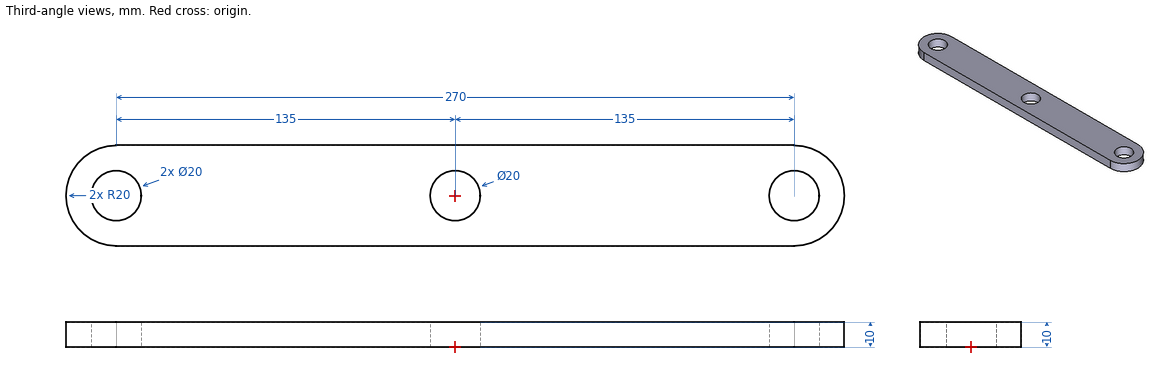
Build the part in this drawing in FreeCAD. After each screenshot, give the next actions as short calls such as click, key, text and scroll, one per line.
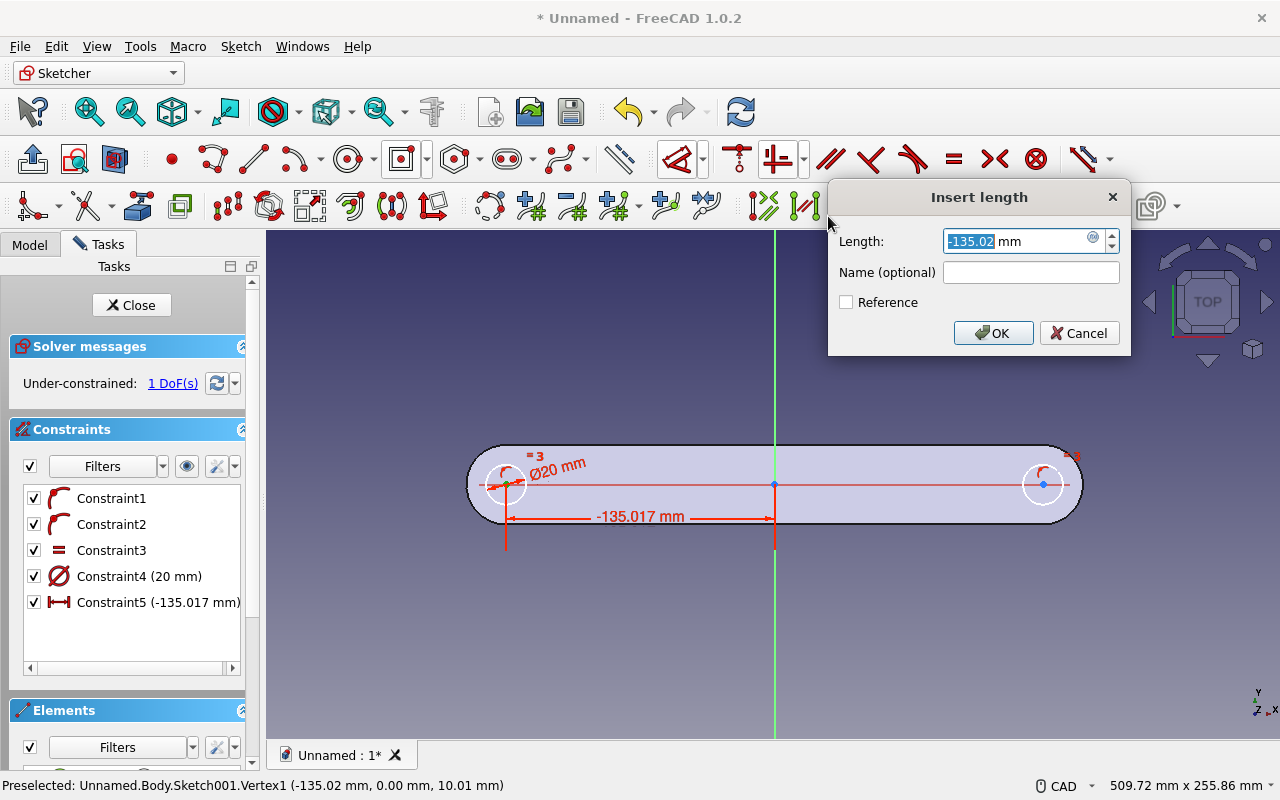
text(-135)
key(Return)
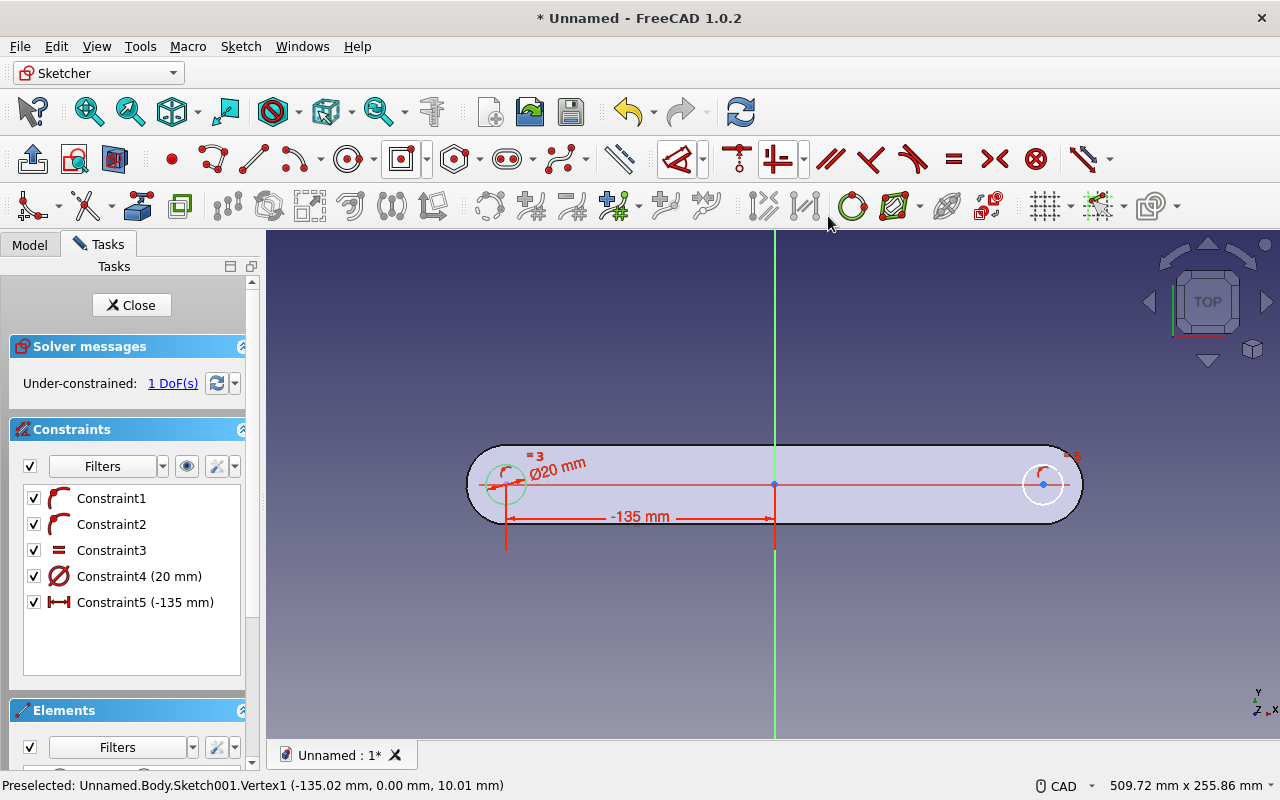
click(1043, 485)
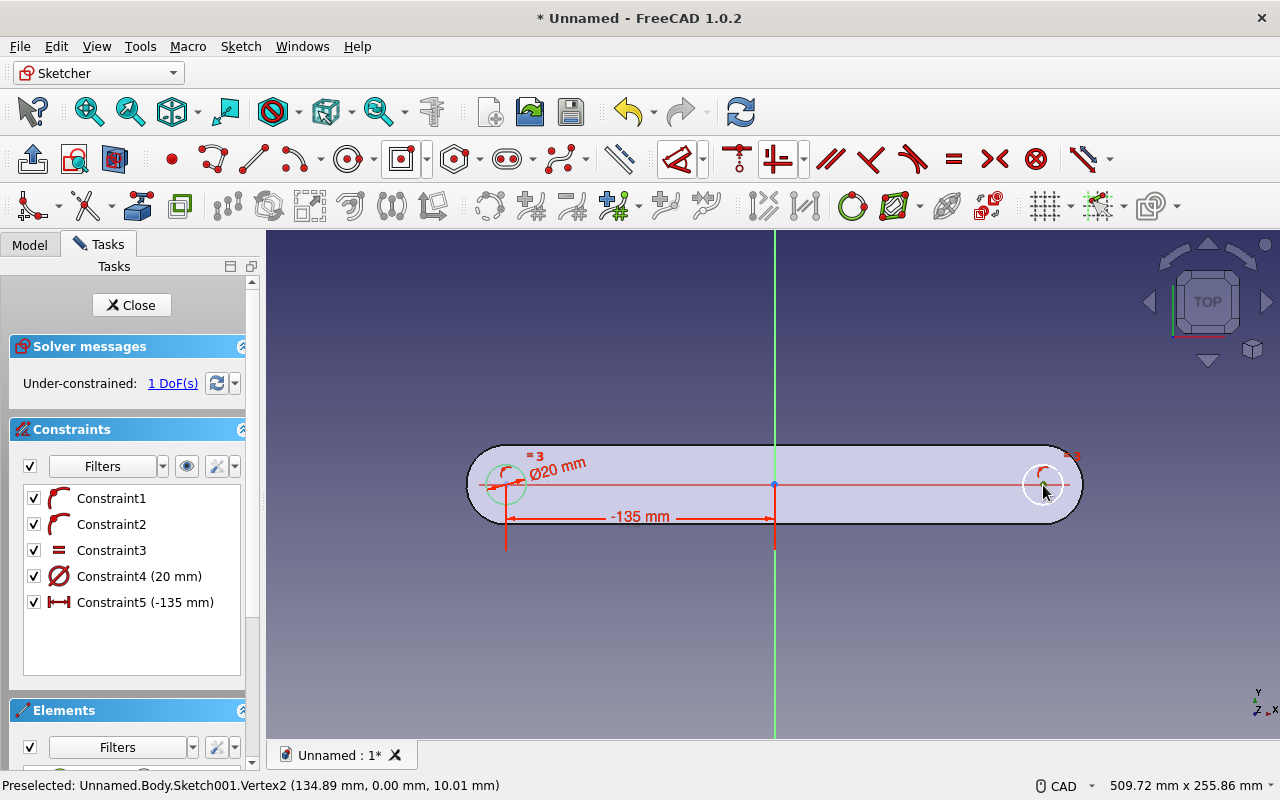
key(l)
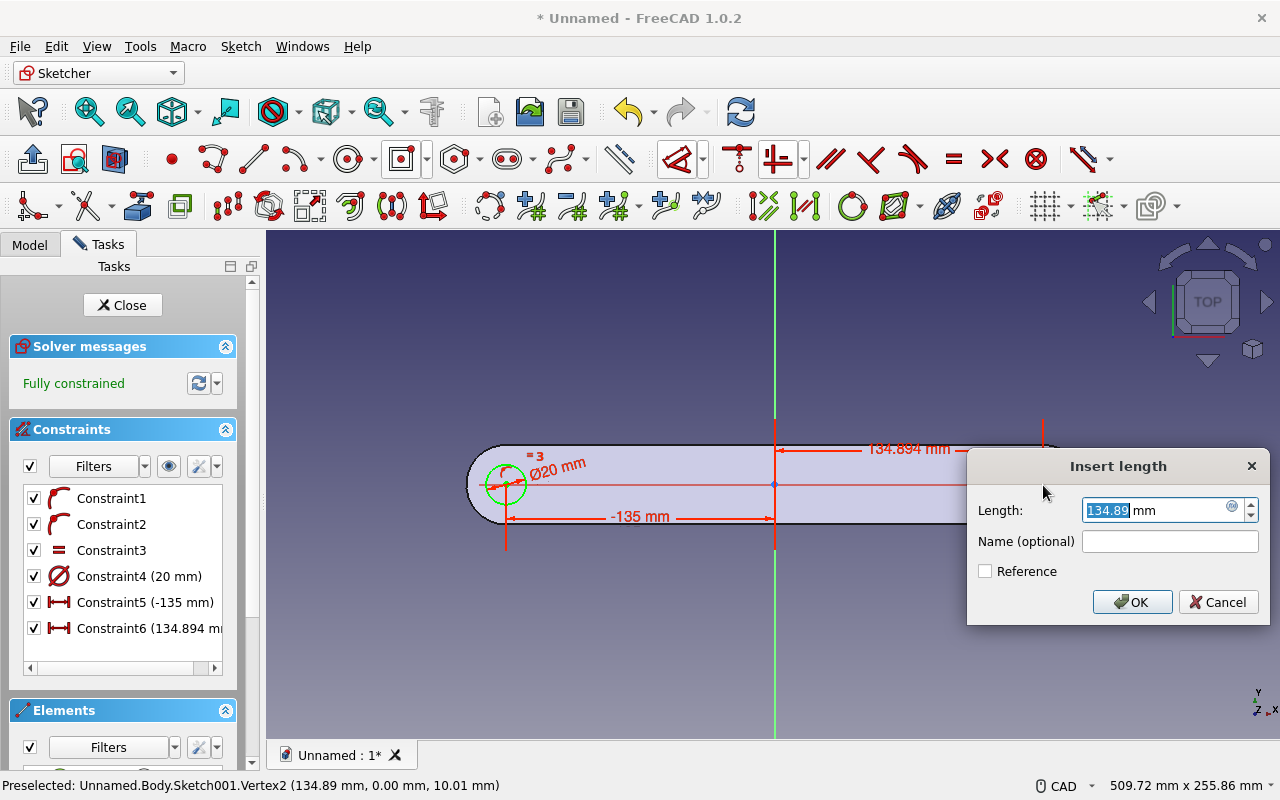
text(135)
key(Return)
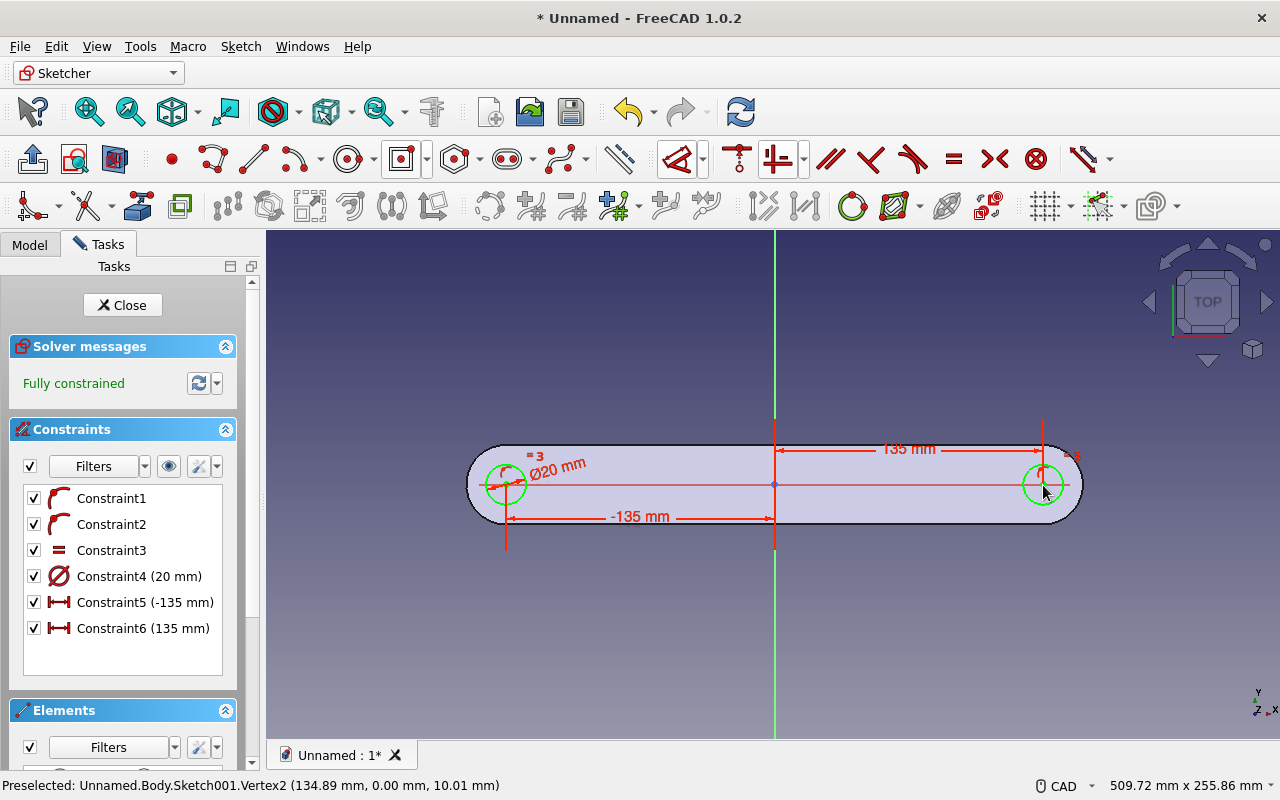
click(123, 305)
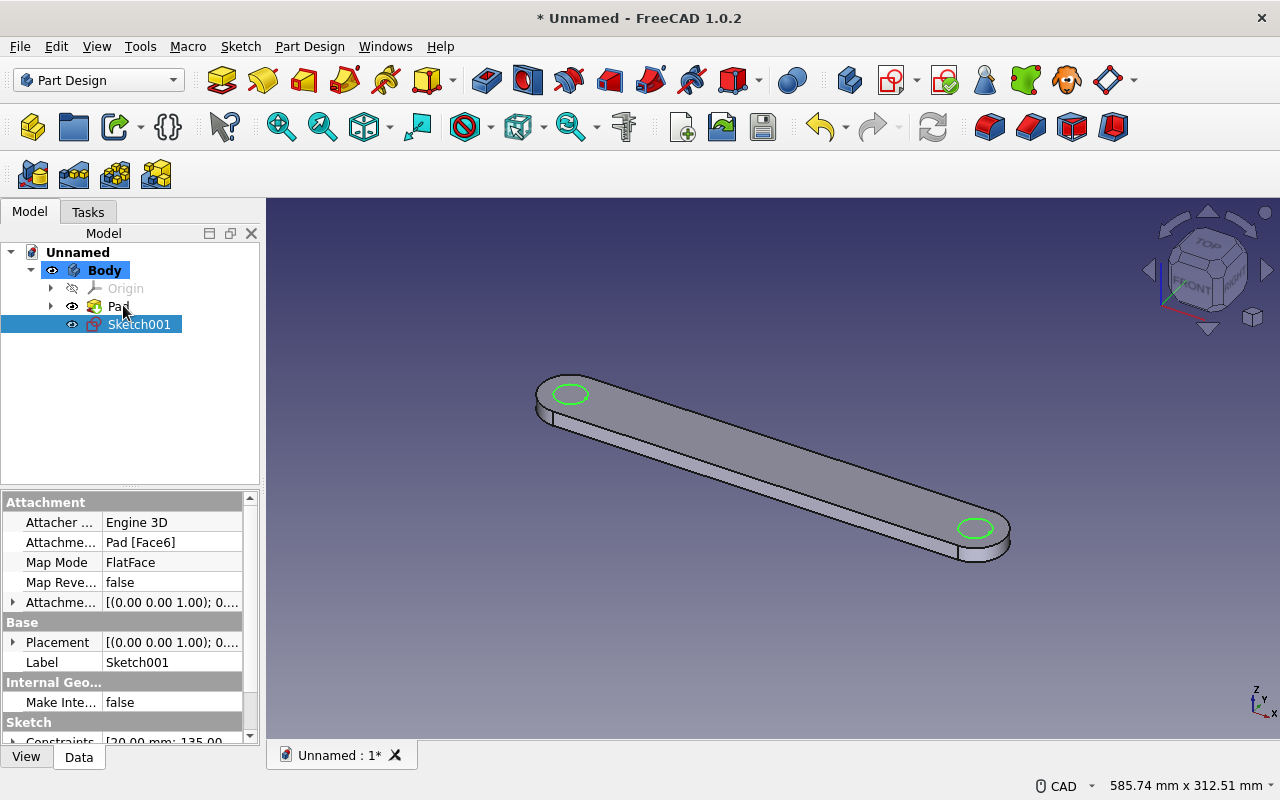
click(487, 80)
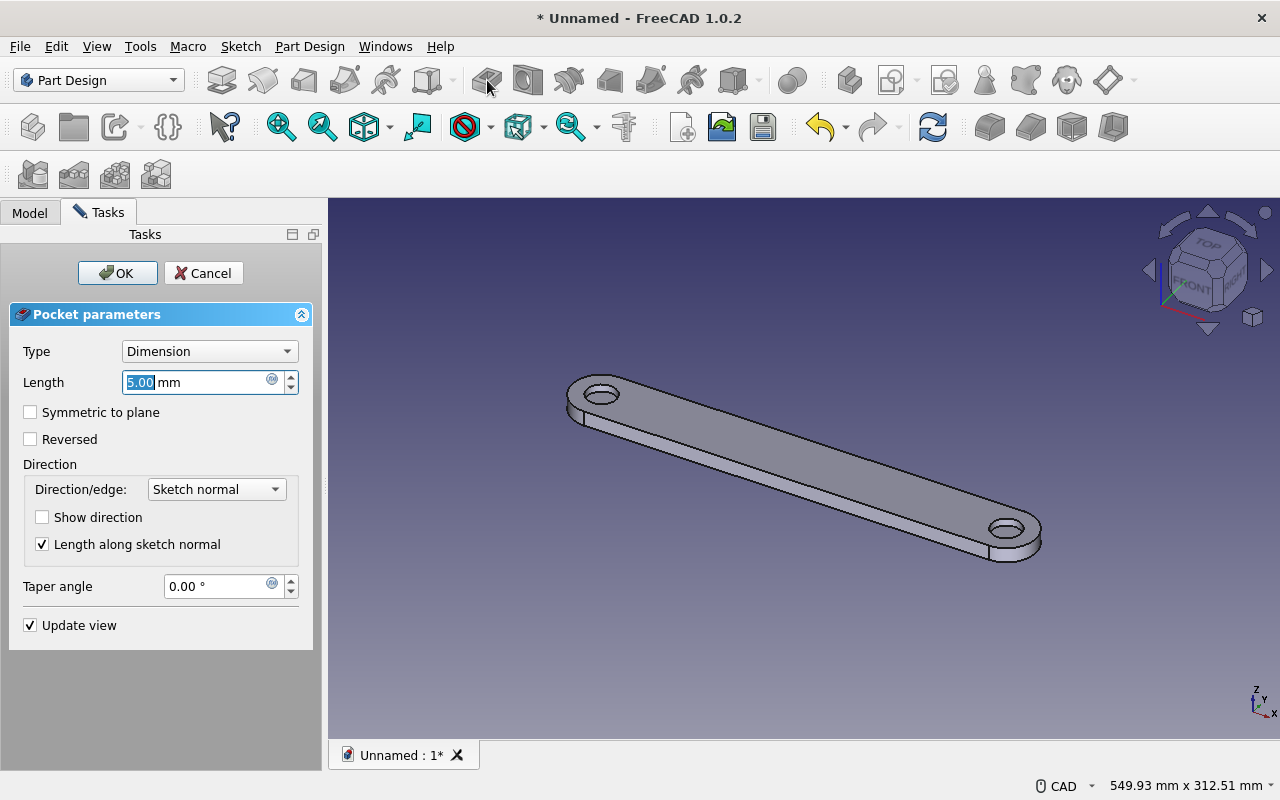
click(210, 352)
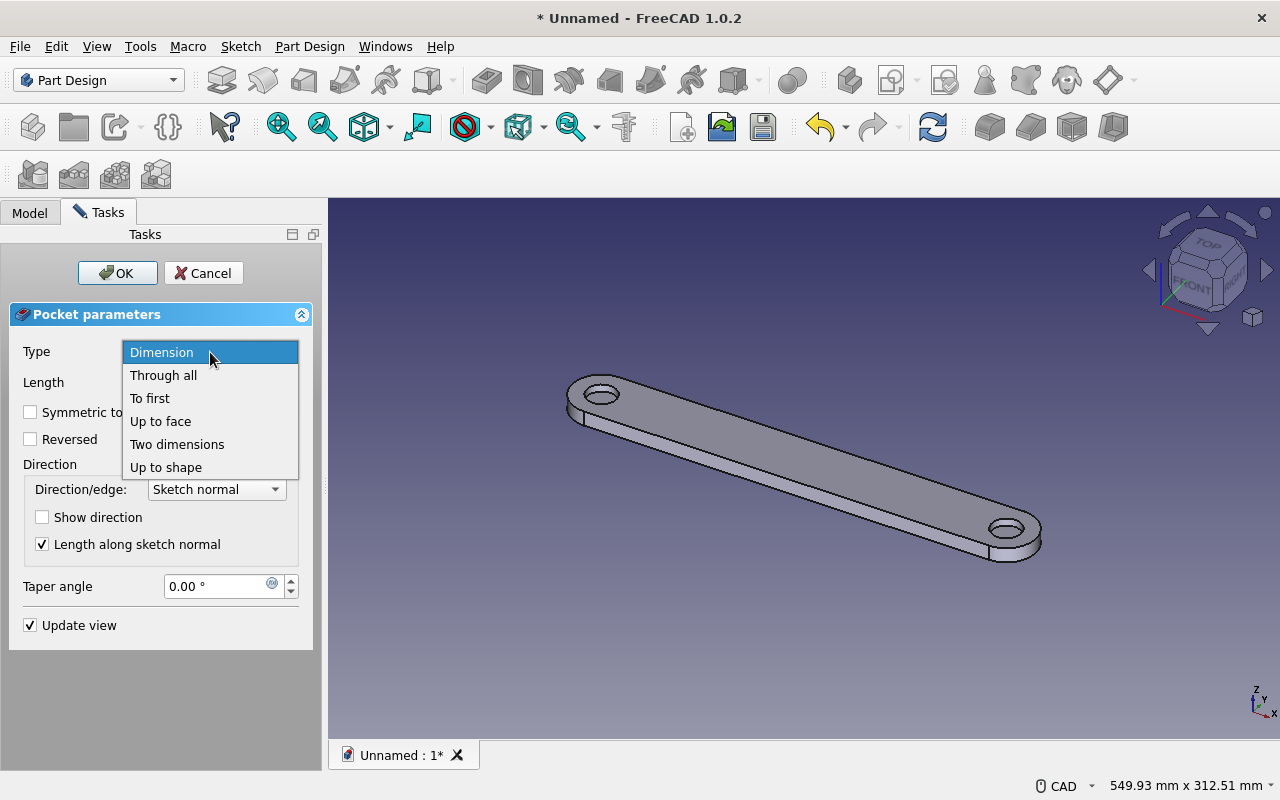
click(208, 376)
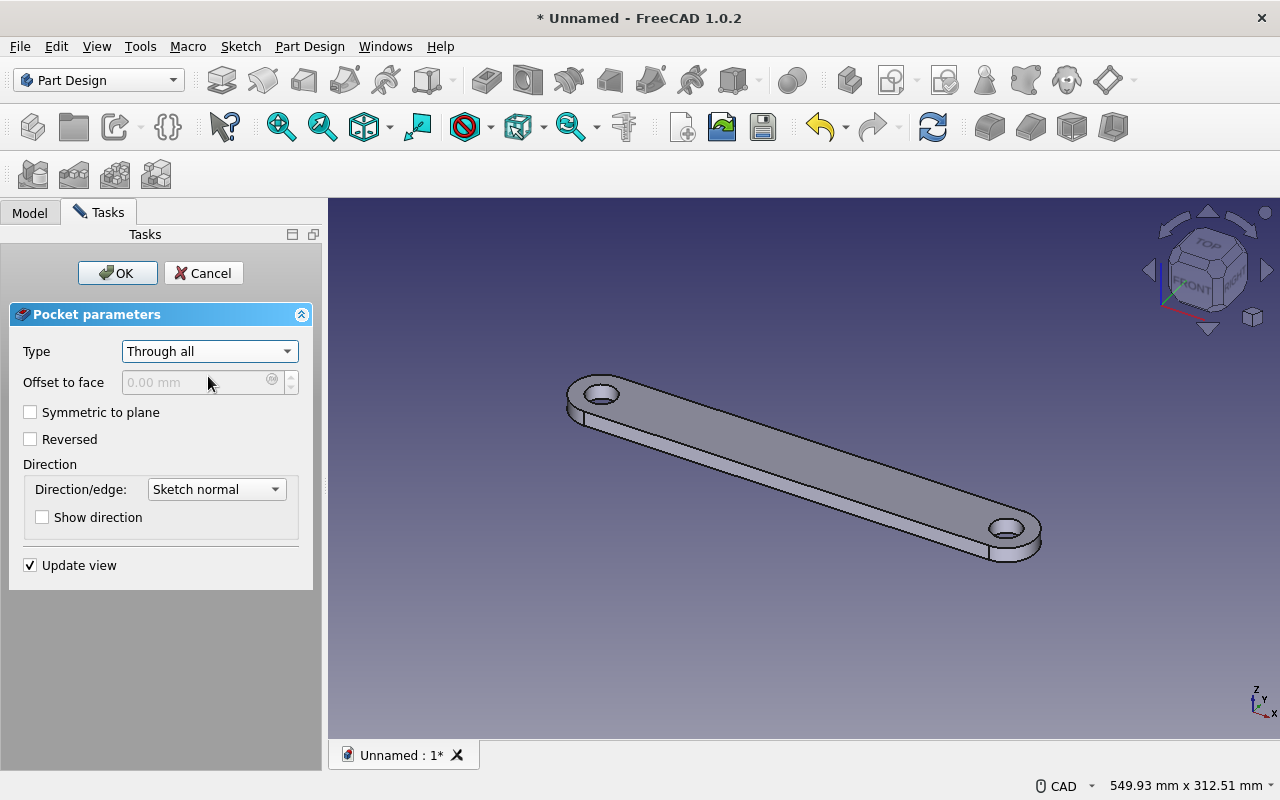
click(118, 273)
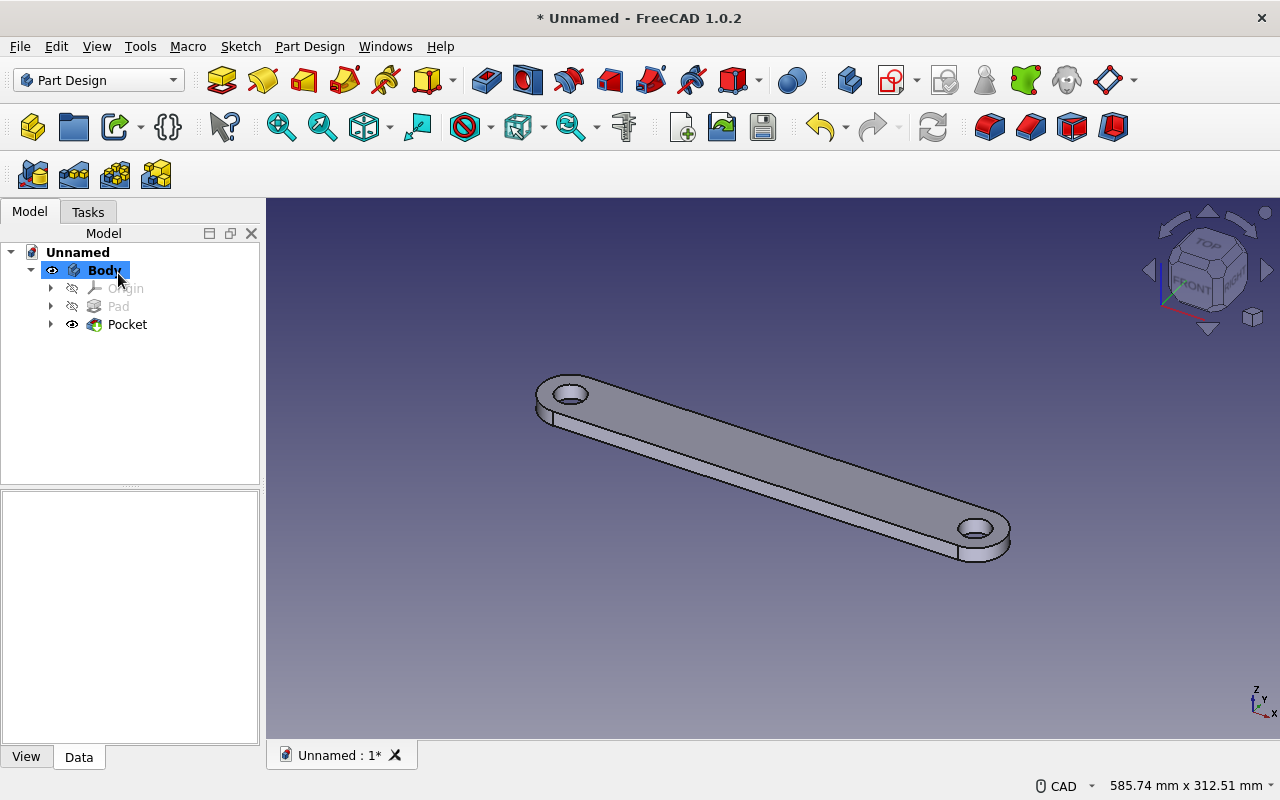
click(906, 504)